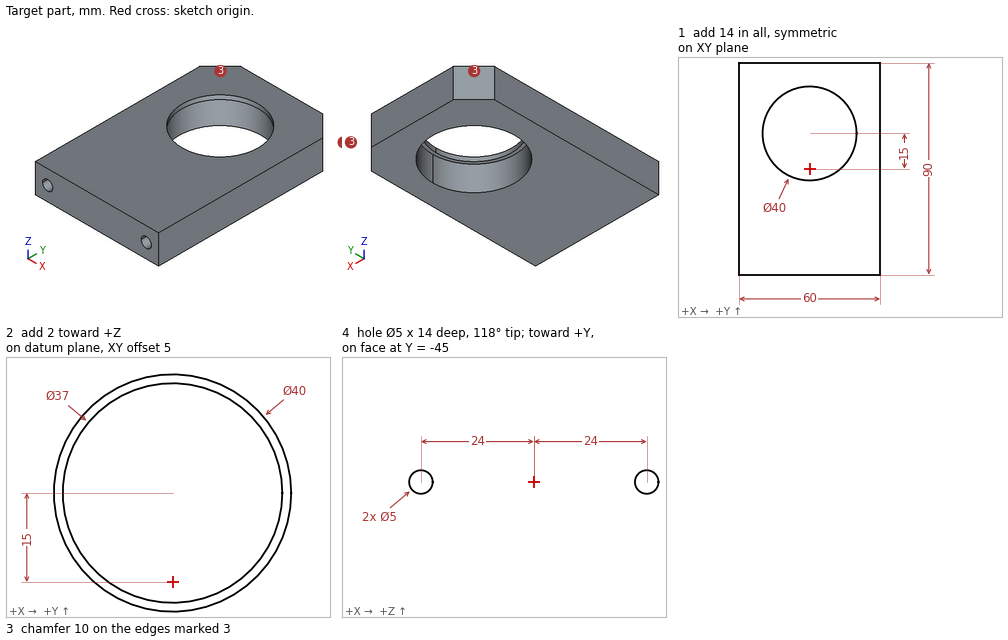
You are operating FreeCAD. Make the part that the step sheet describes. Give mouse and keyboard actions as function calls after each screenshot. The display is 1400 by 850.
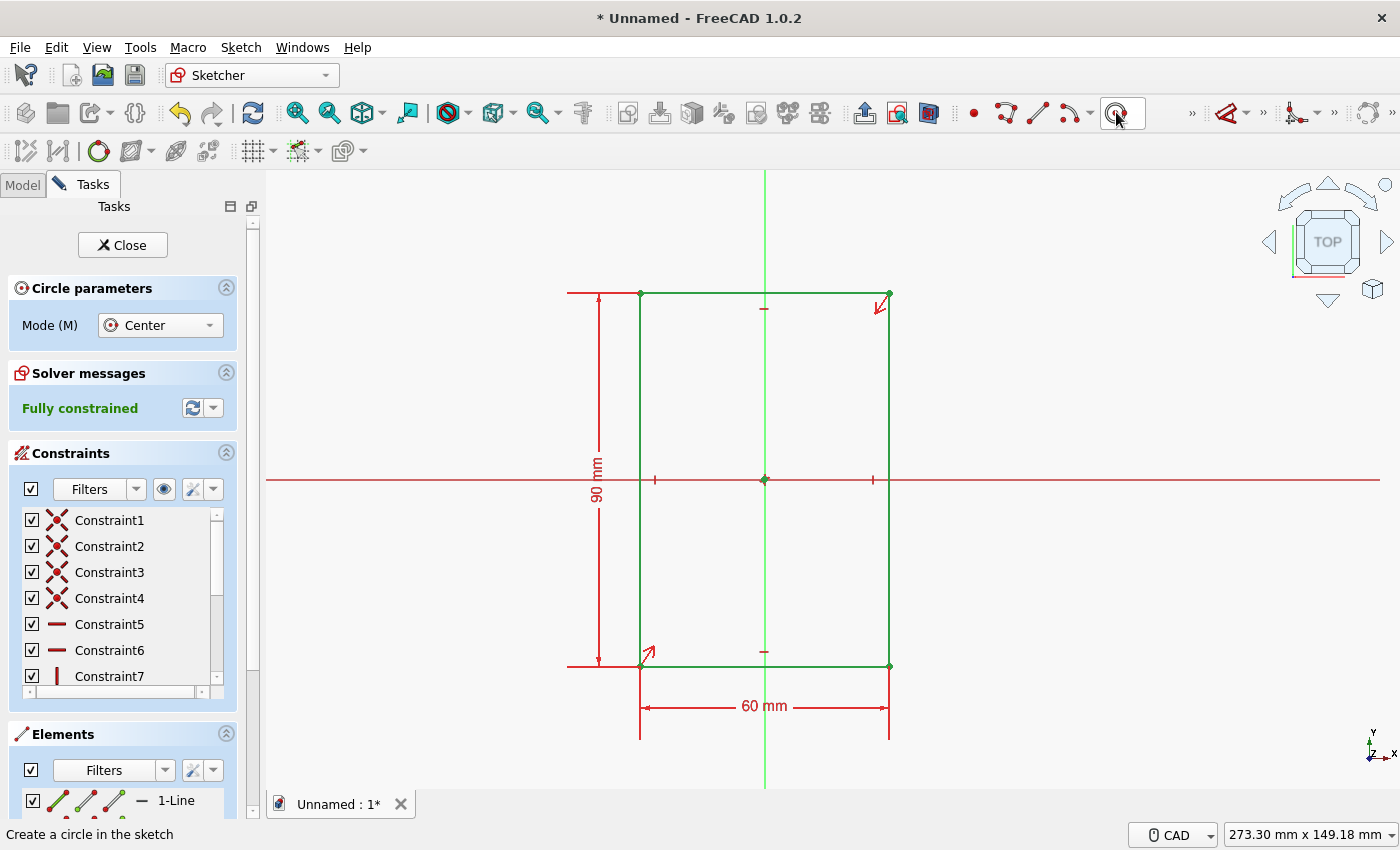
click(765, 418)
move(823, 359)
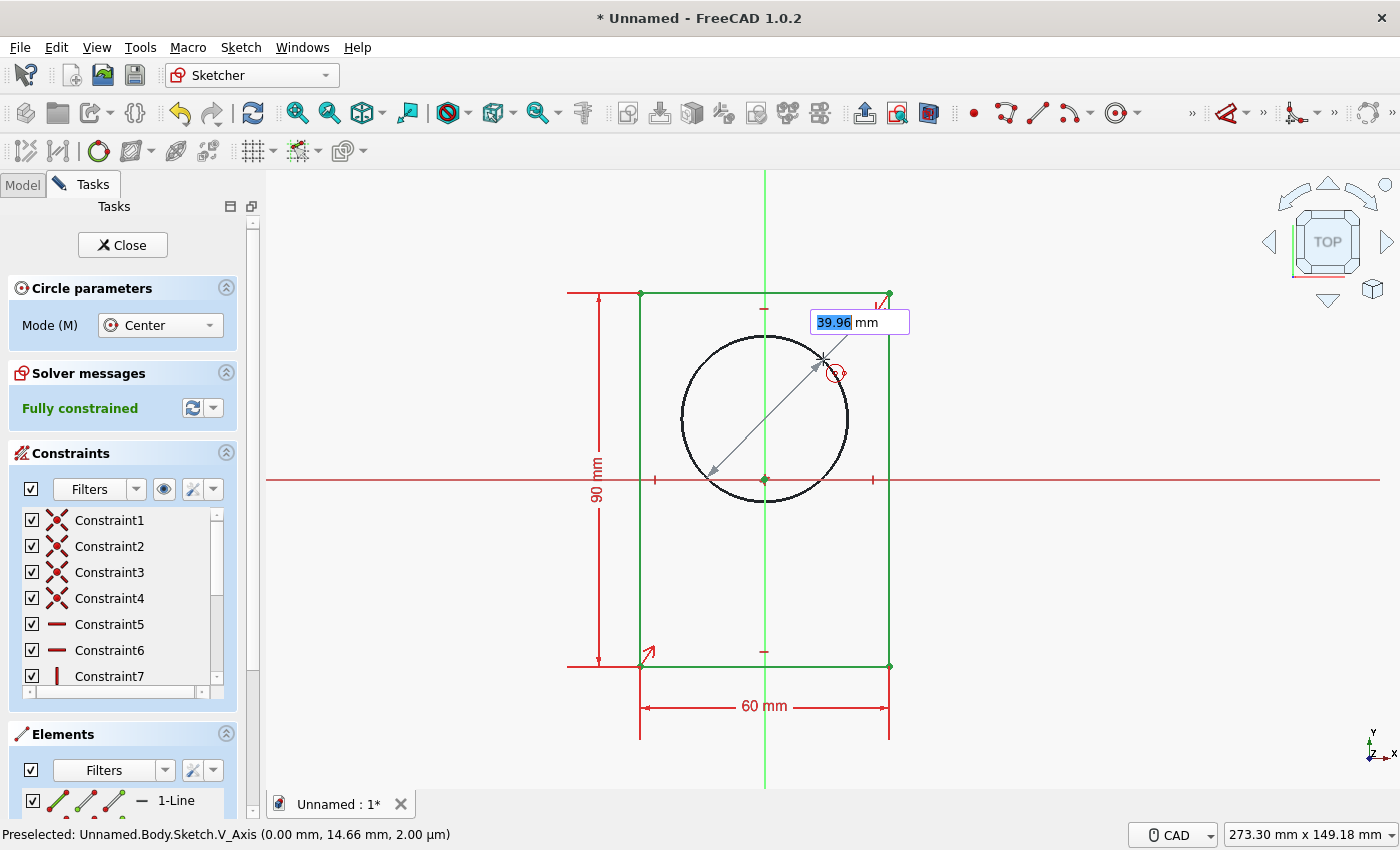
text(40)
key(Return)
key(Escape)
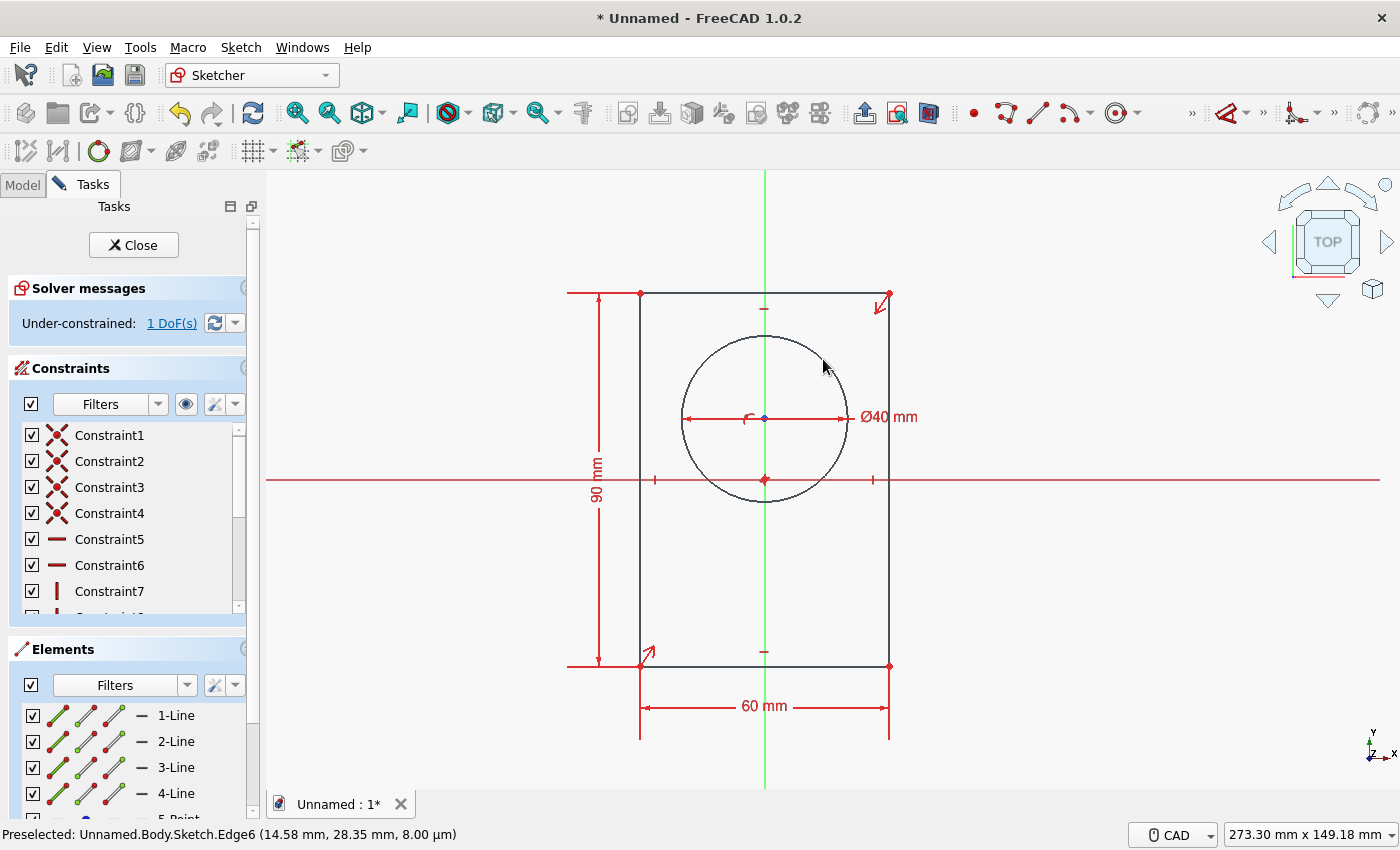
click(1226, 114)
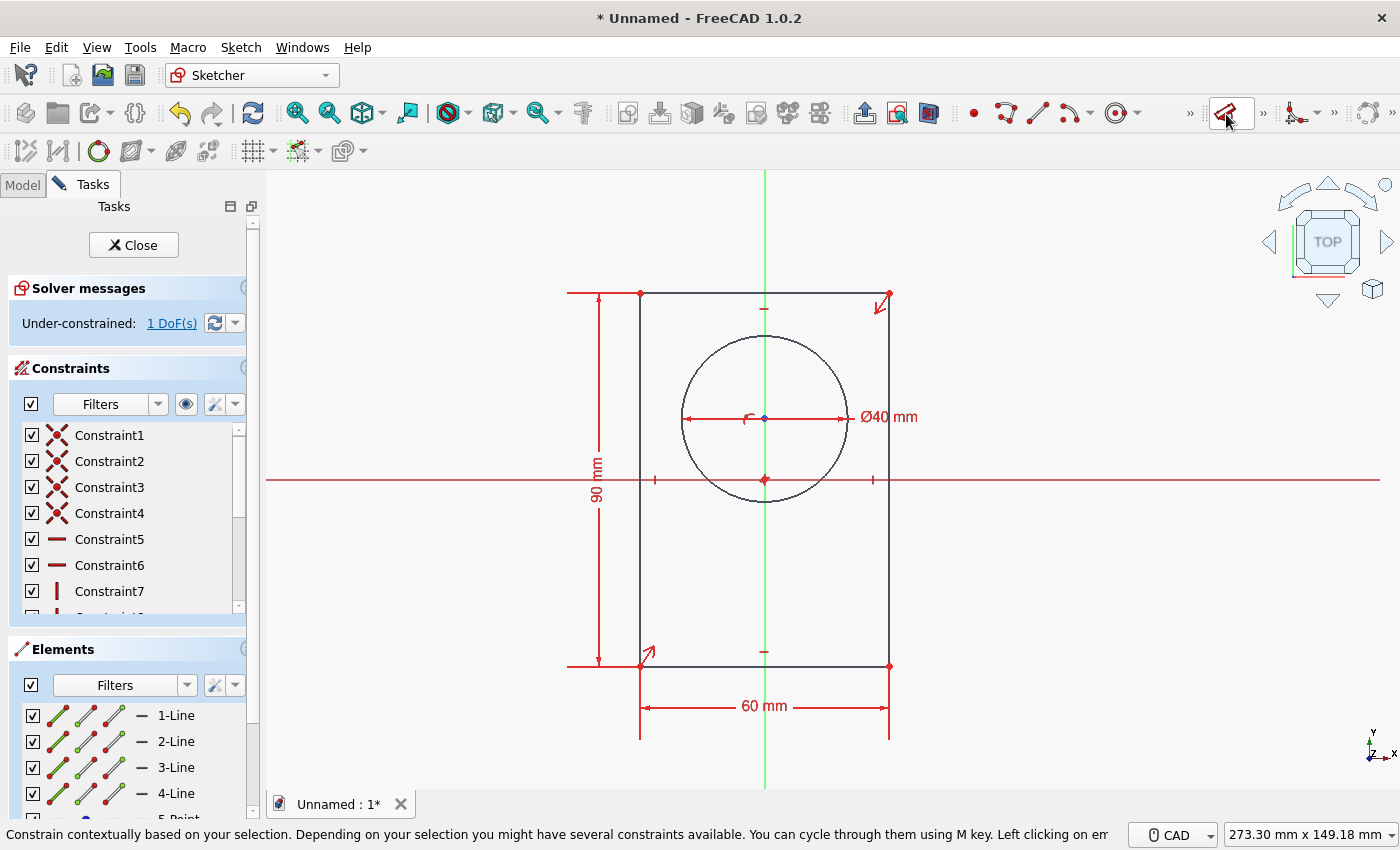
click(765, 419)
click(799, 449)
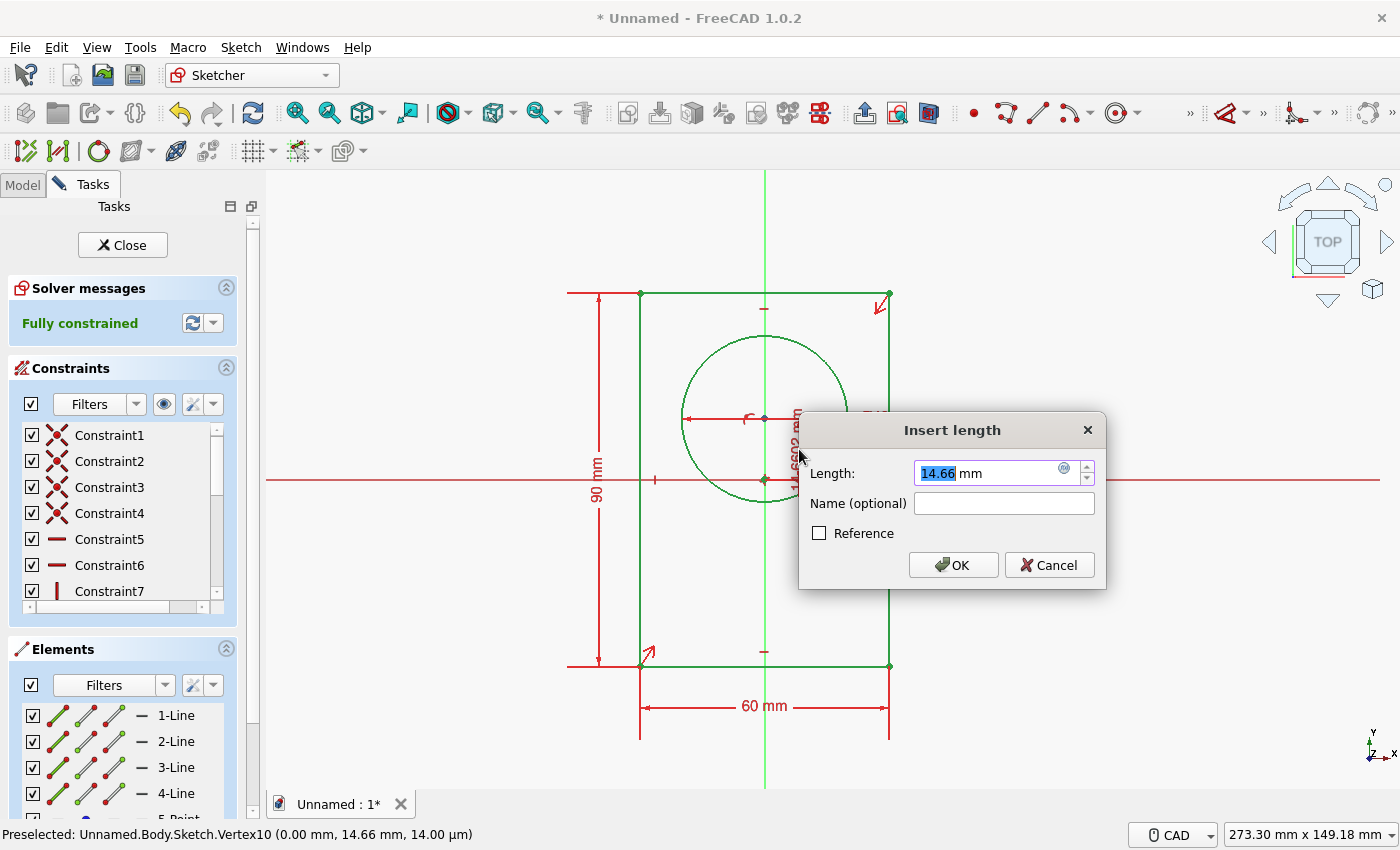
text(15)
key(Return)
key(Escape)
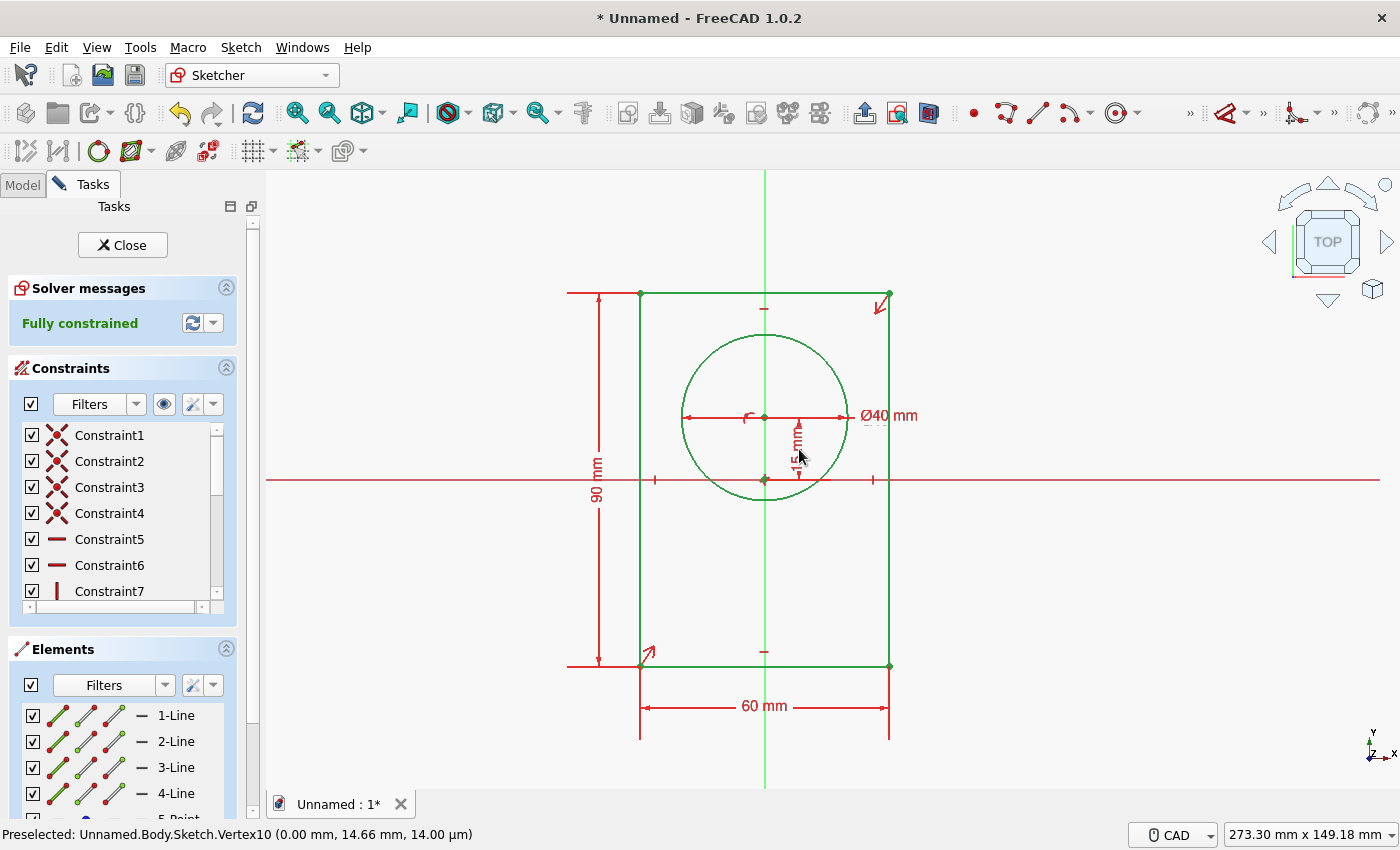
click(123, 245)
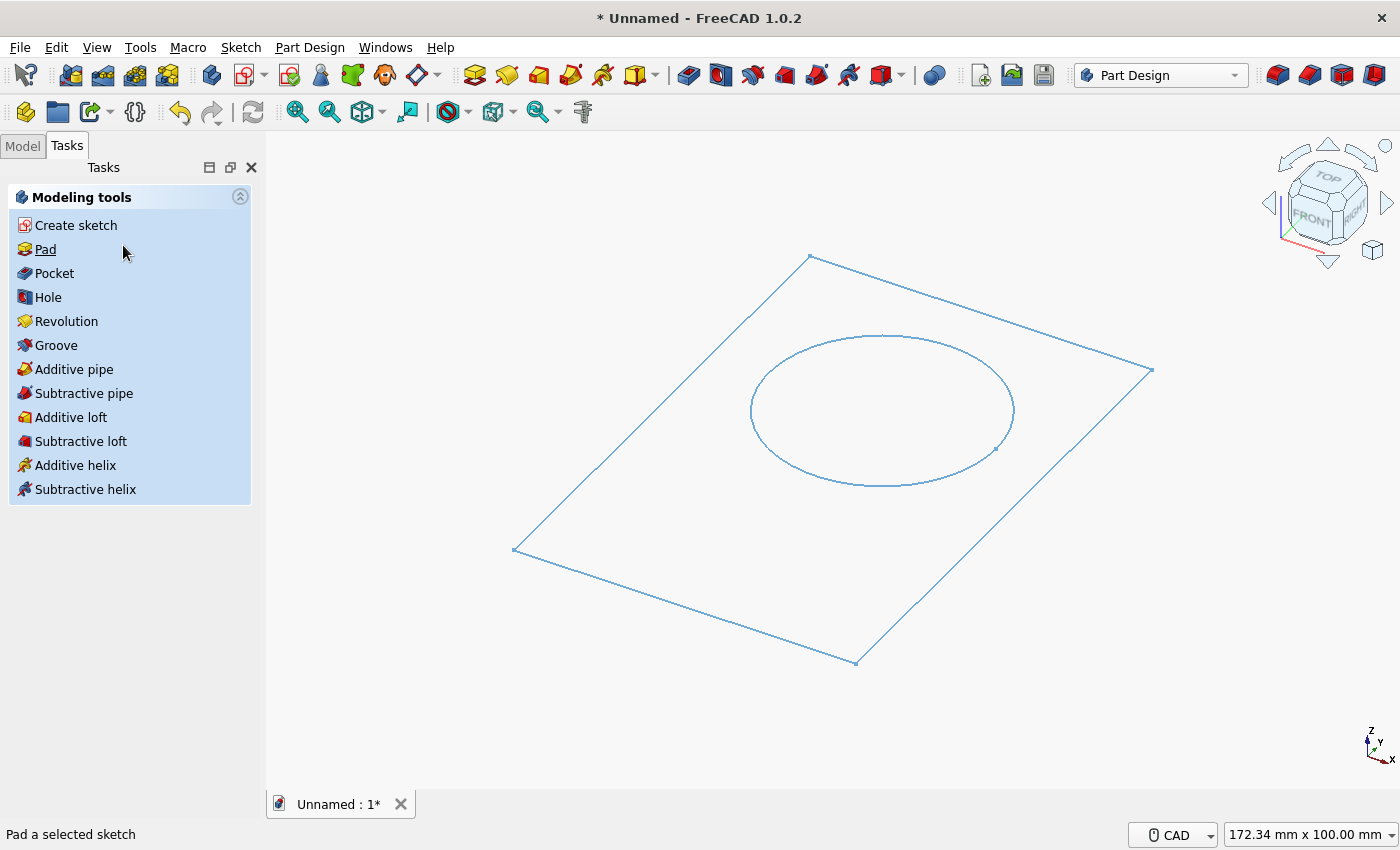
click(476, 76)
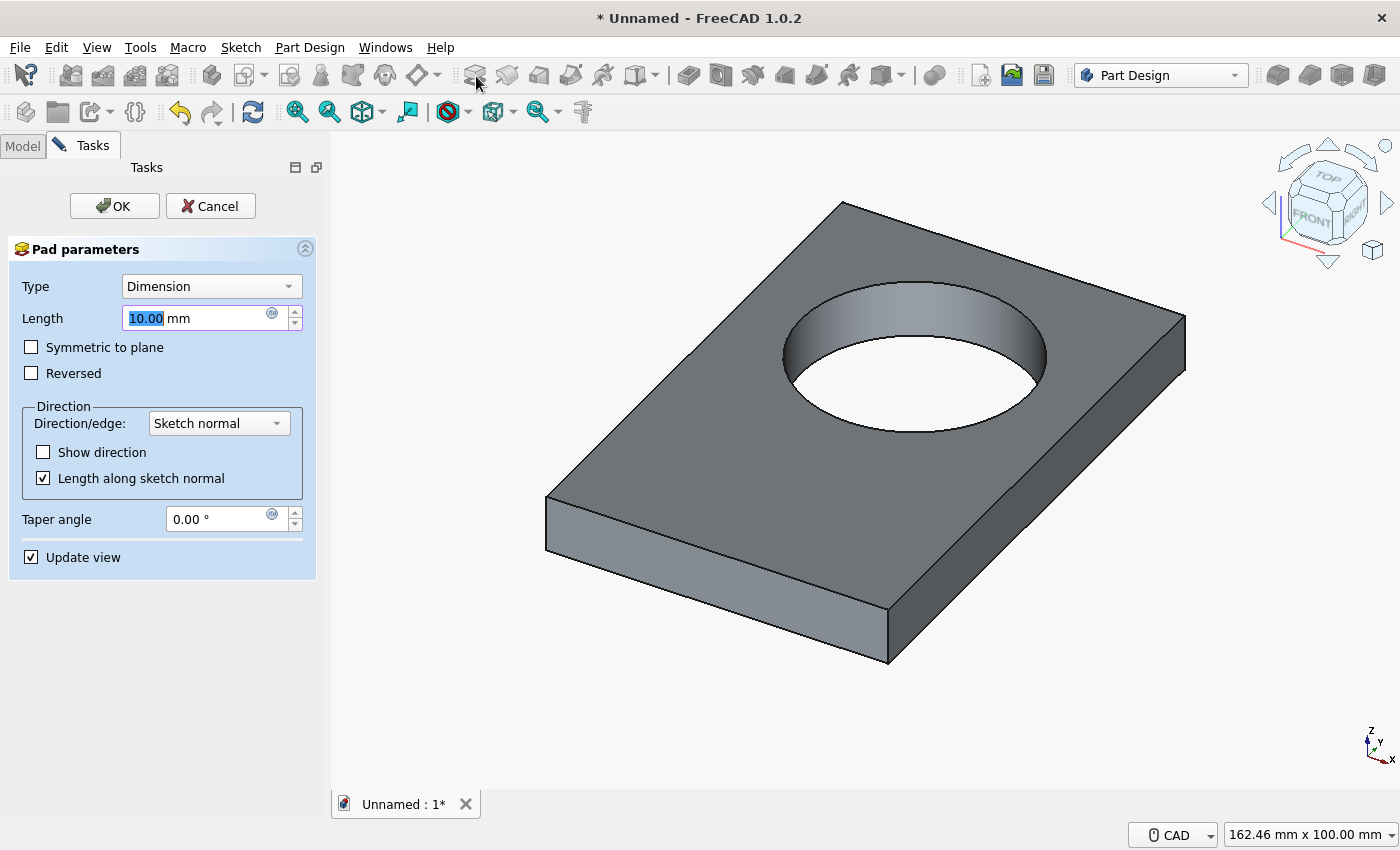
text(14)
key(Tab)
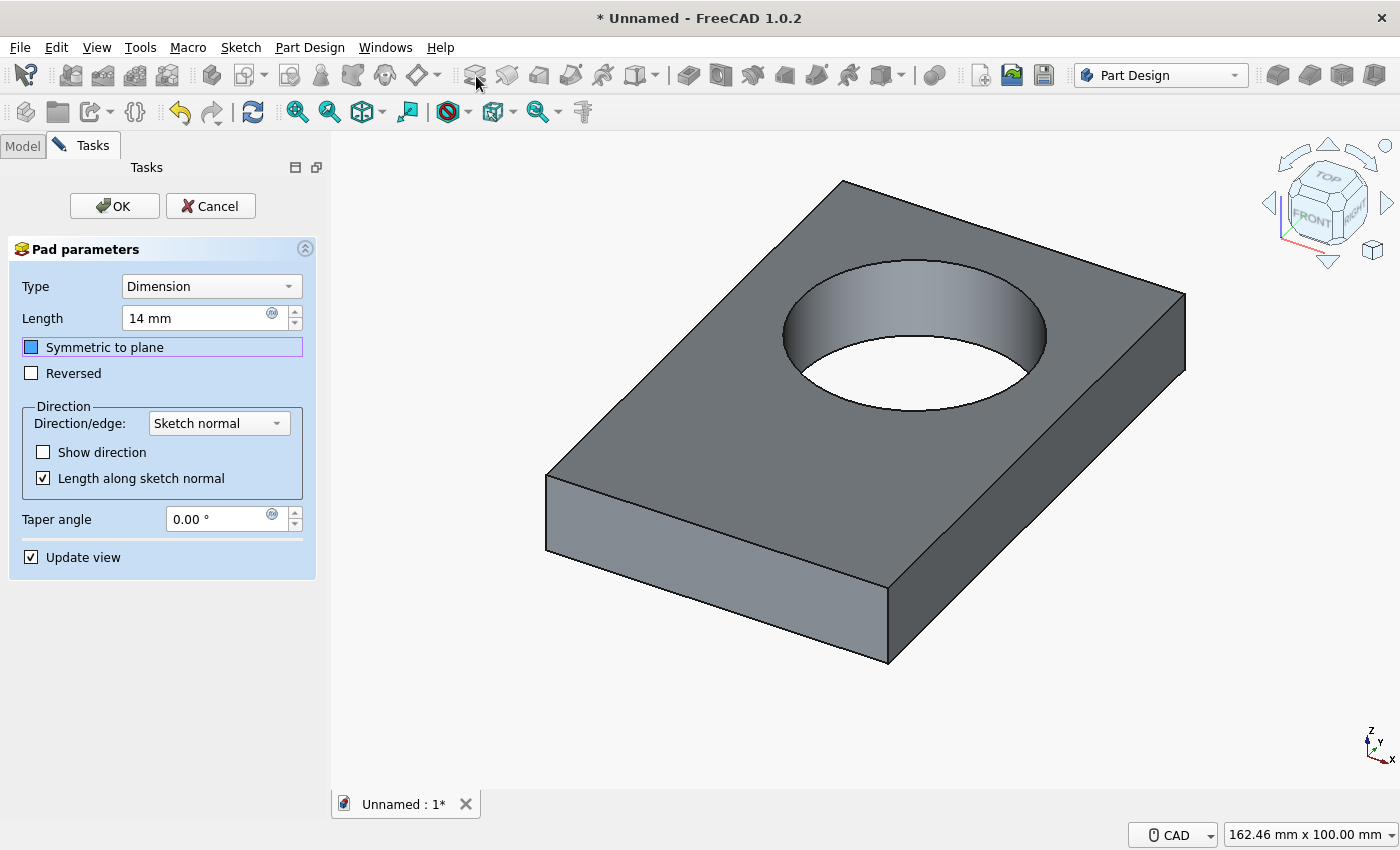
click(30, 347)